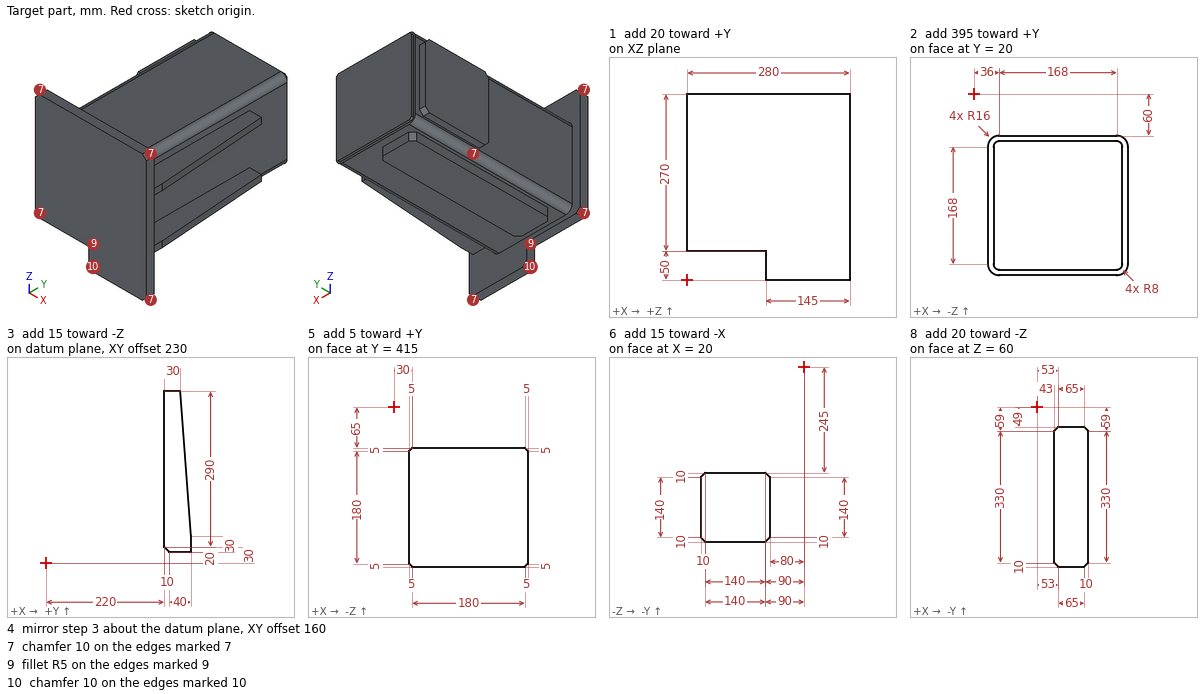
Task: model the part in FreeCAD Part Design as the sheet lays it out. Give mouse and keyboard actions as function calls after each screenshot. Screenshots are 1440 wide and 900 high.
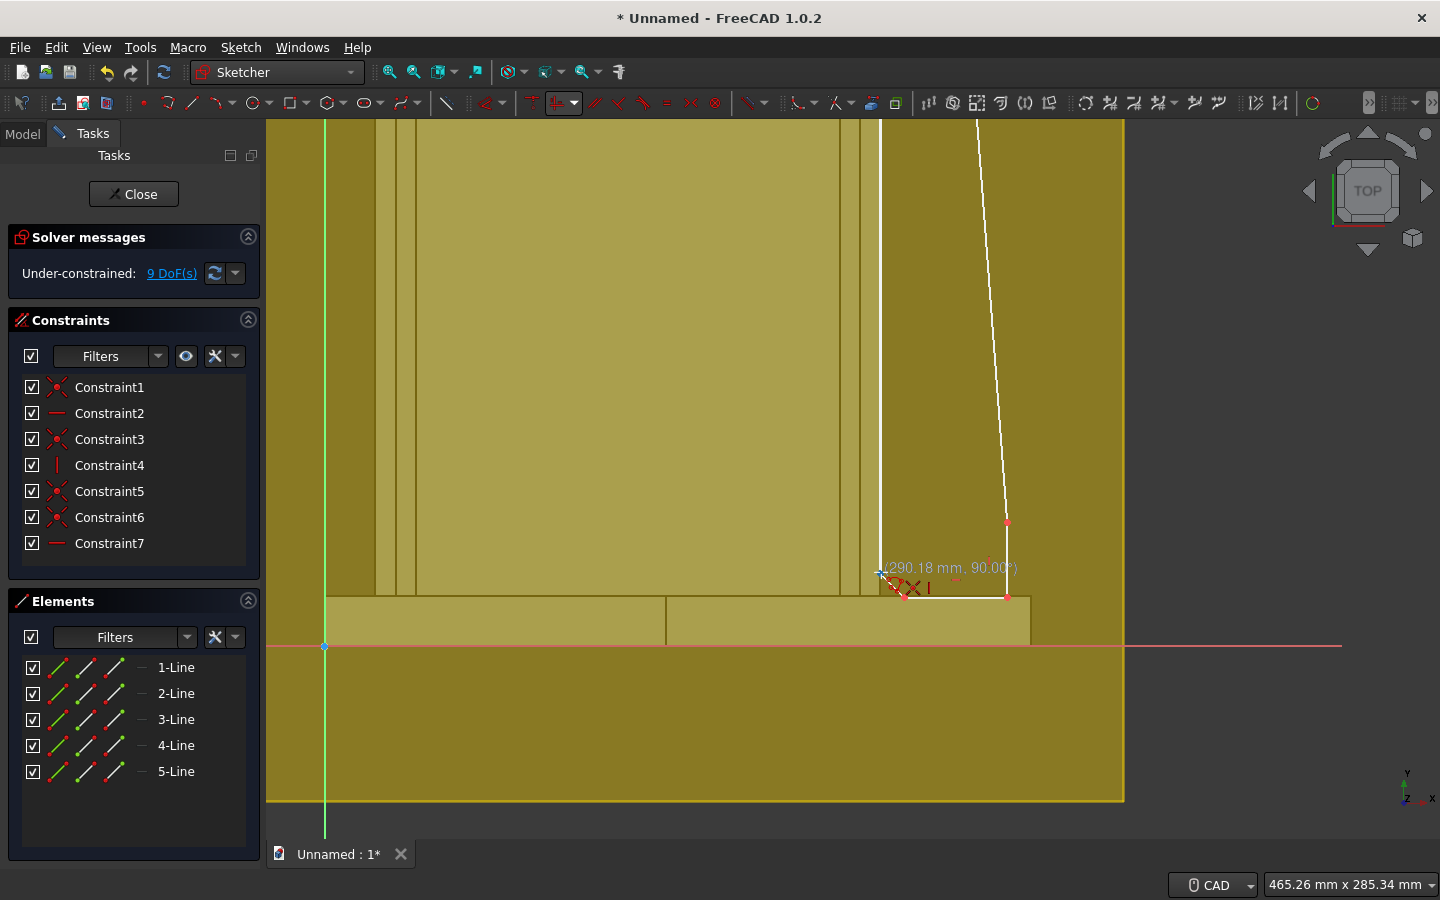
click(880, 573)
key(Escape)
key(Escape)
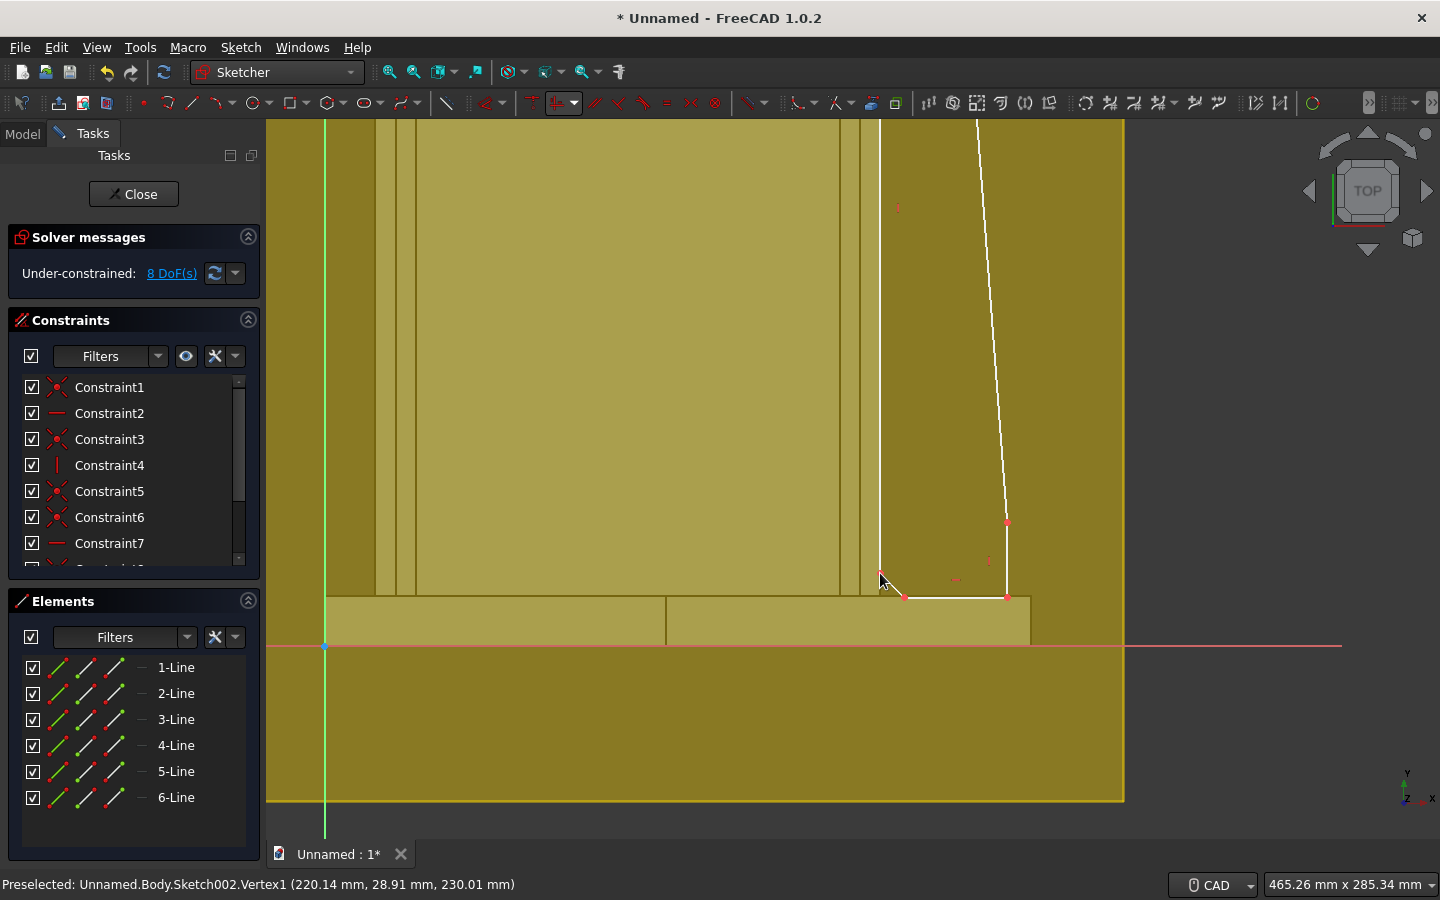
click(486, 104)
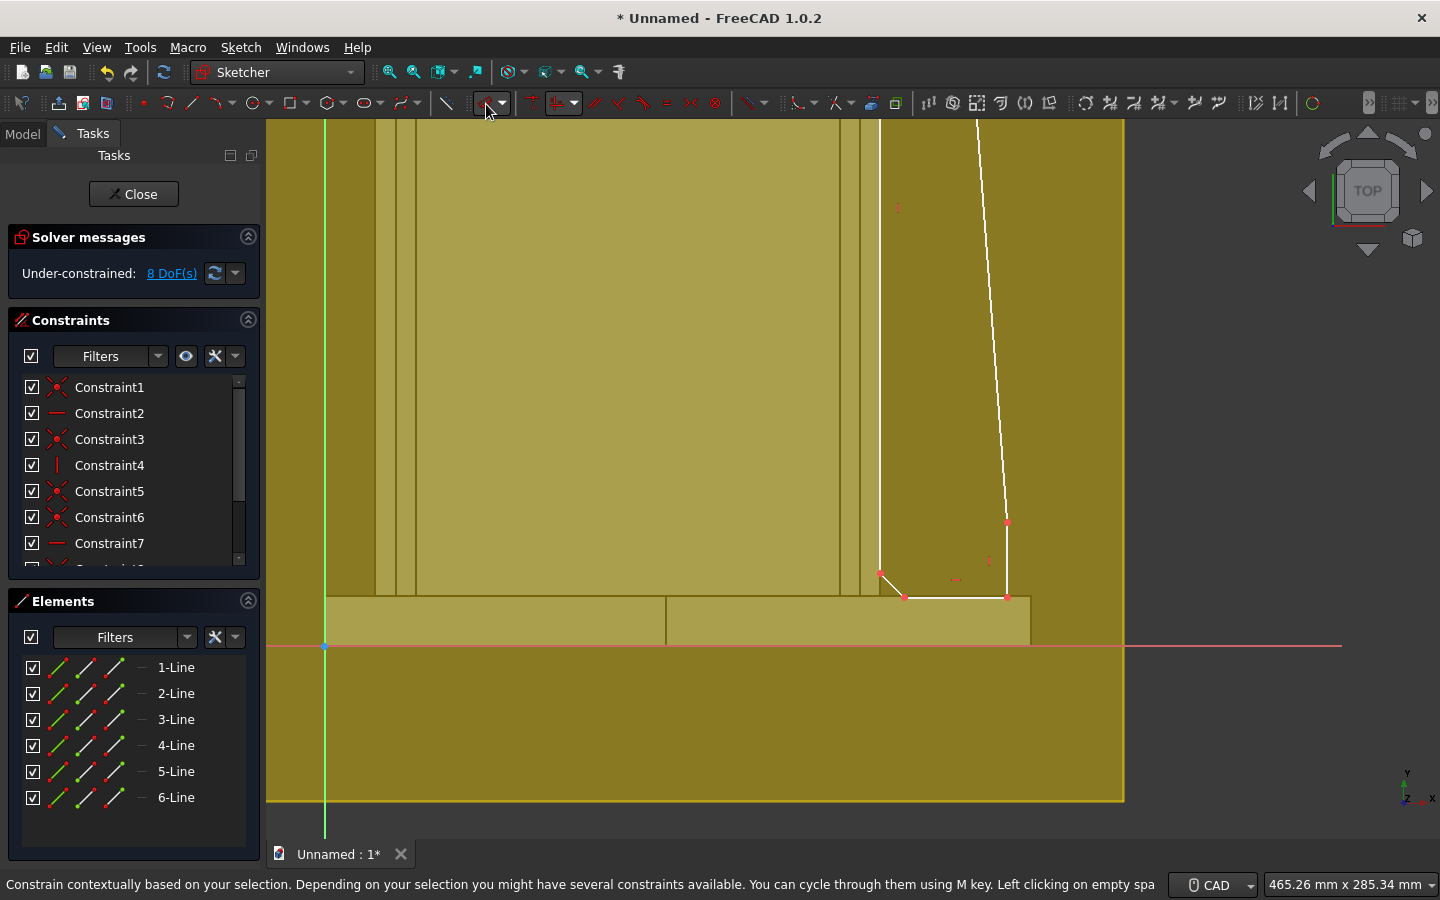
click(936, 598)
click(956, 632)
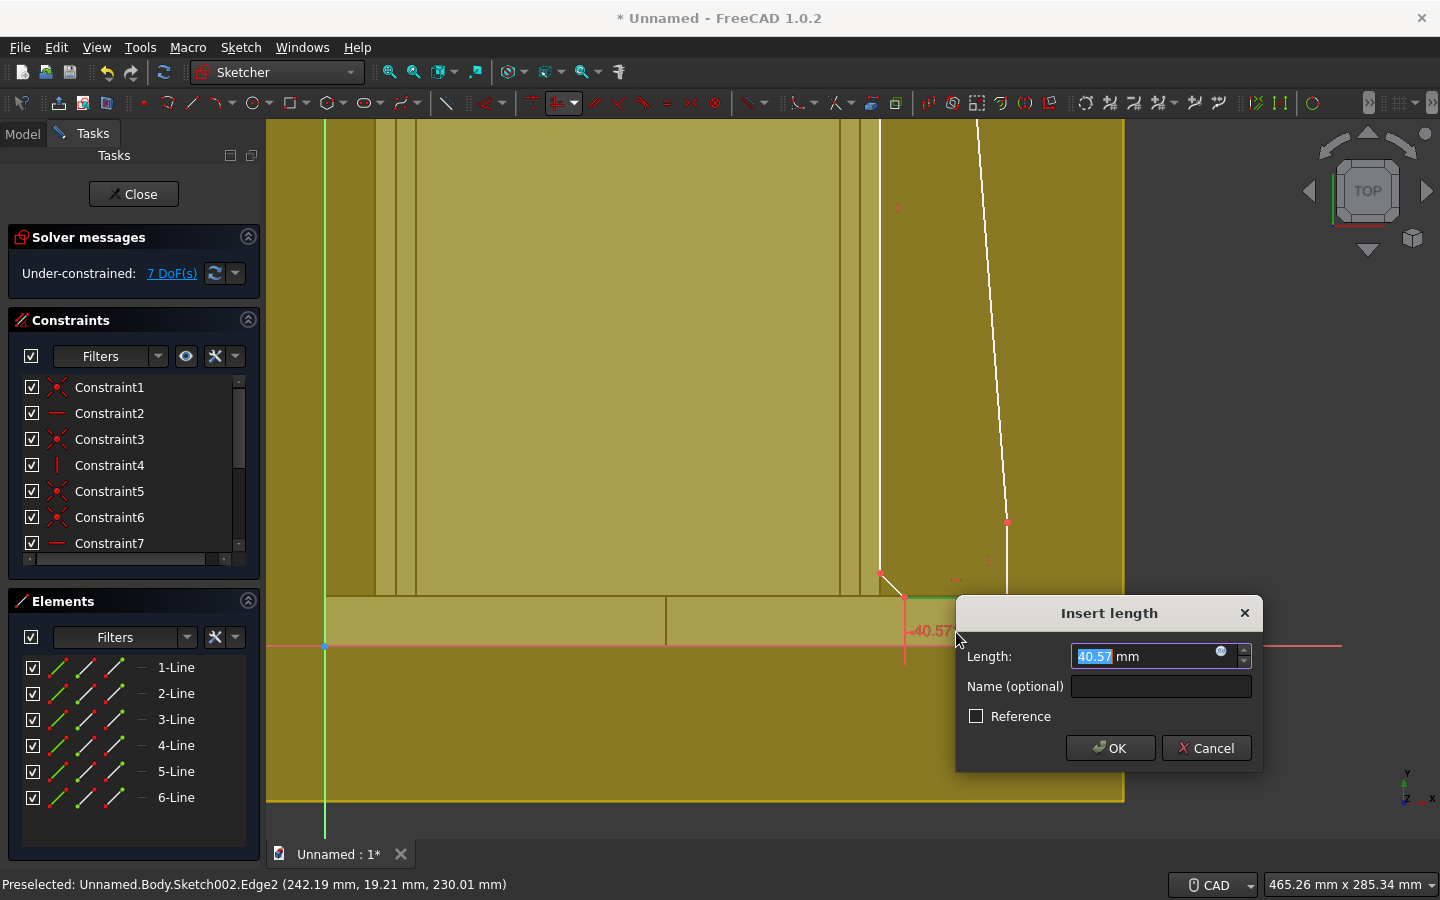
text(40)
key(Return)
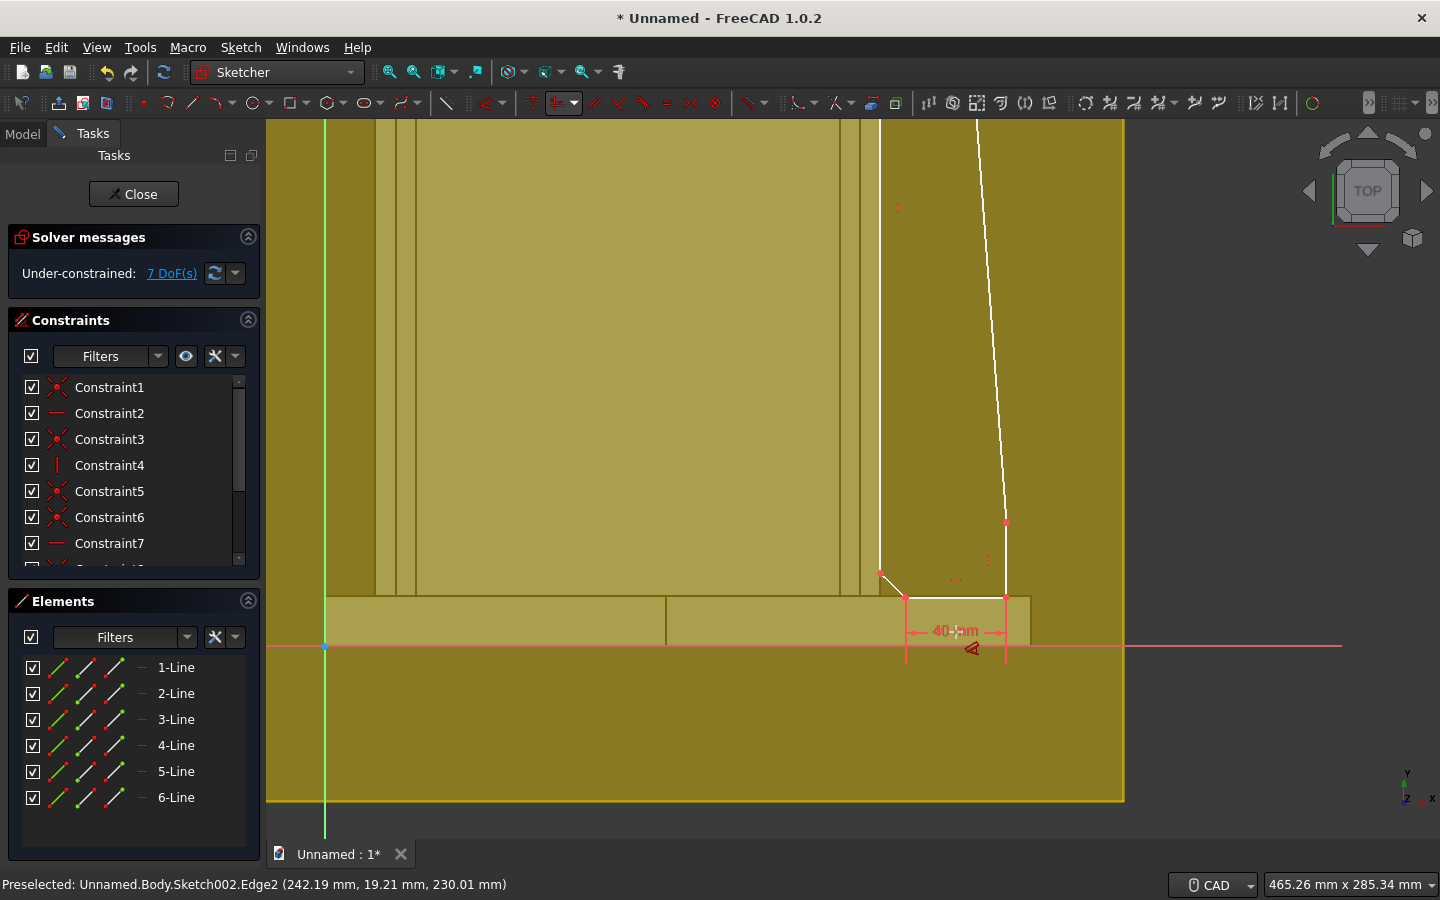
click(1006, 575)
click(1040, 560)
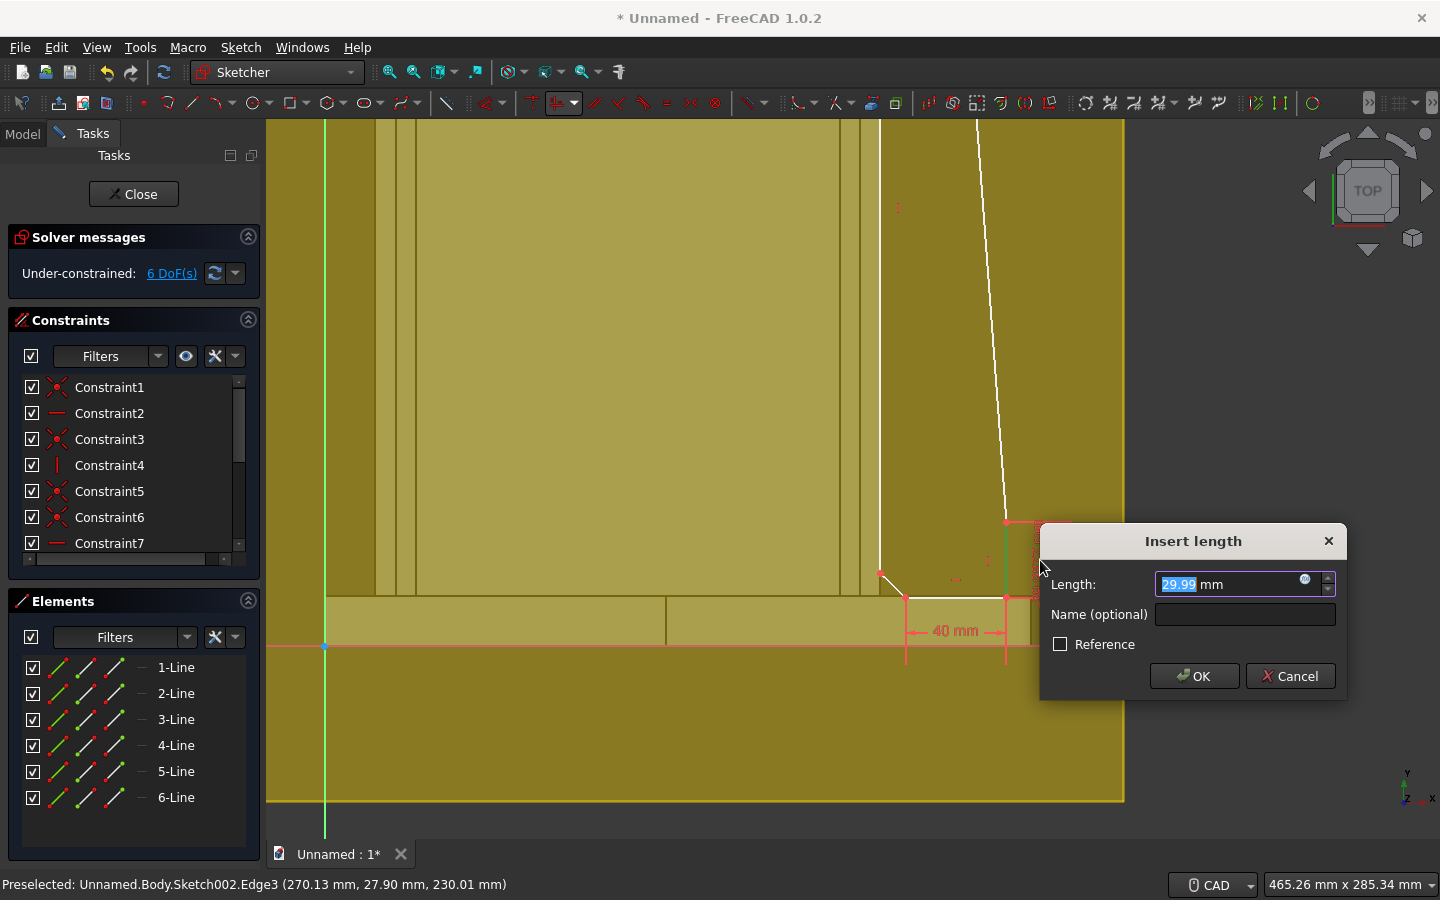
text(30)
key(Return)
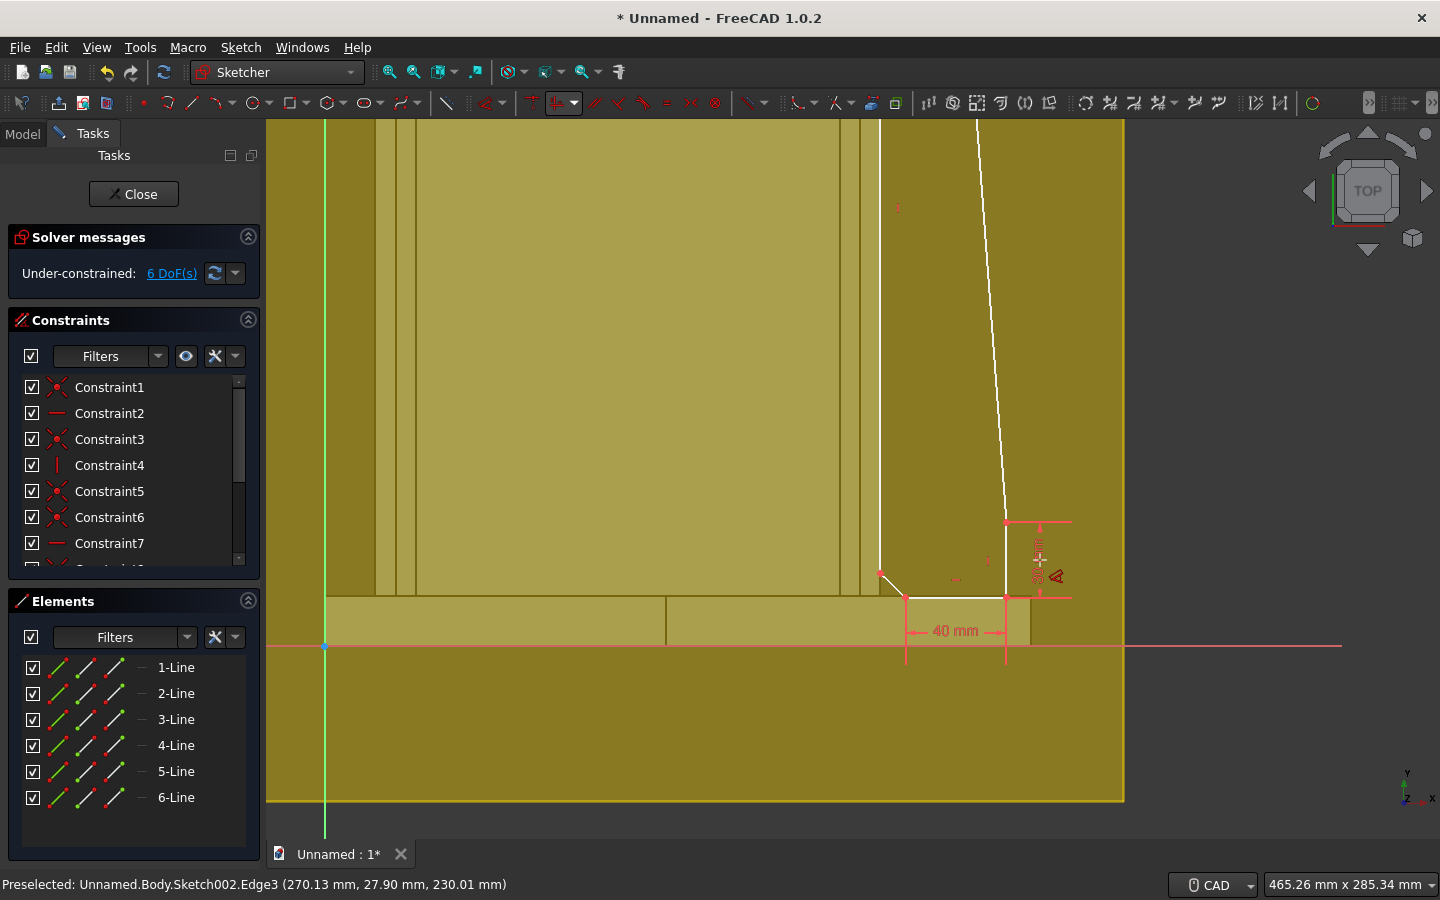
scroll(929, 766, down, 3)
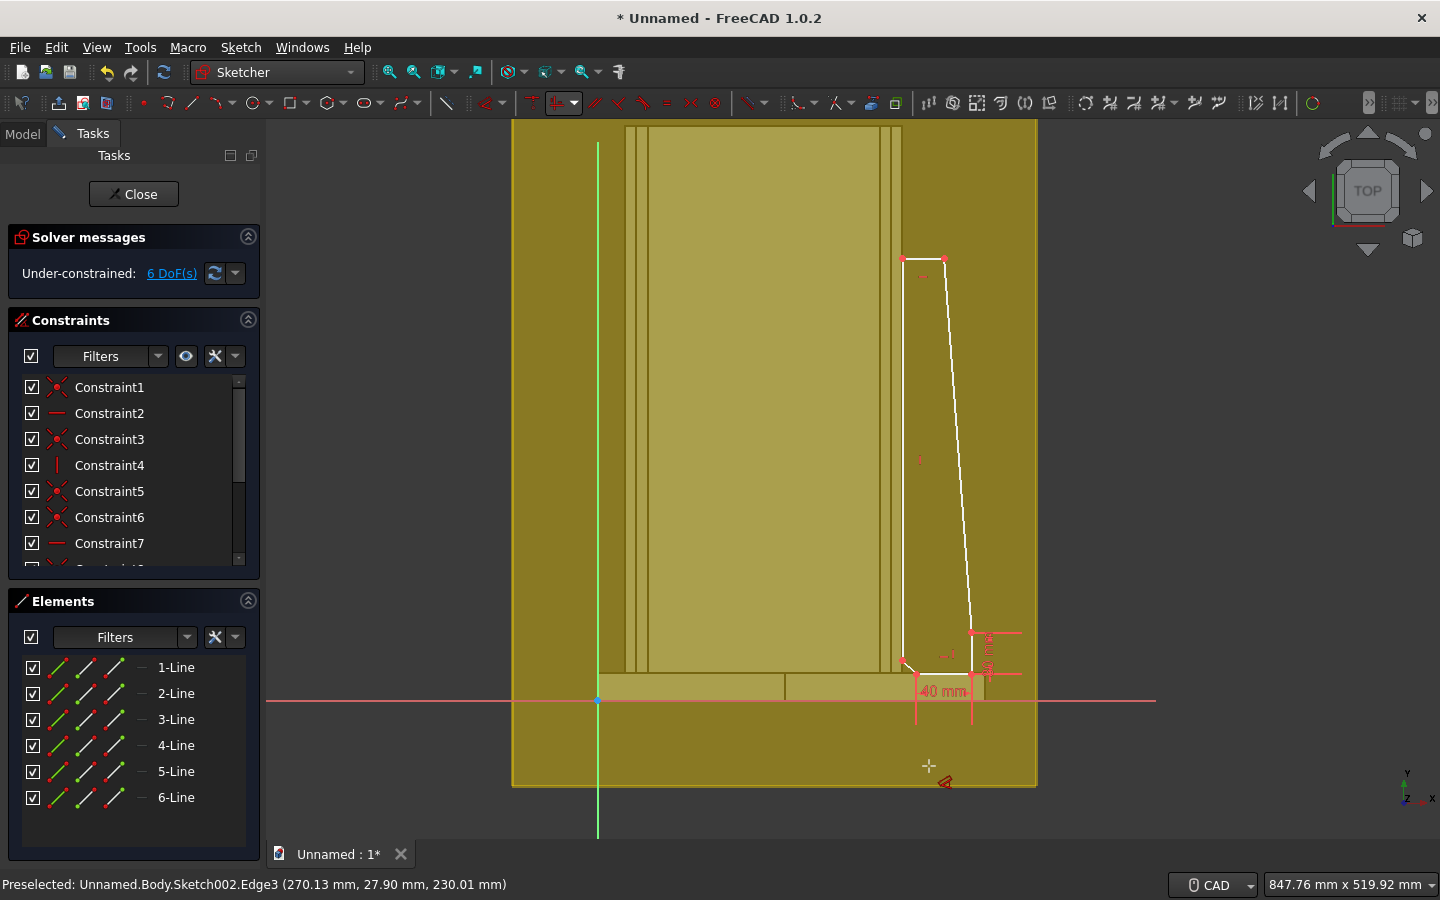
click(932, 259)
click(923, 225)